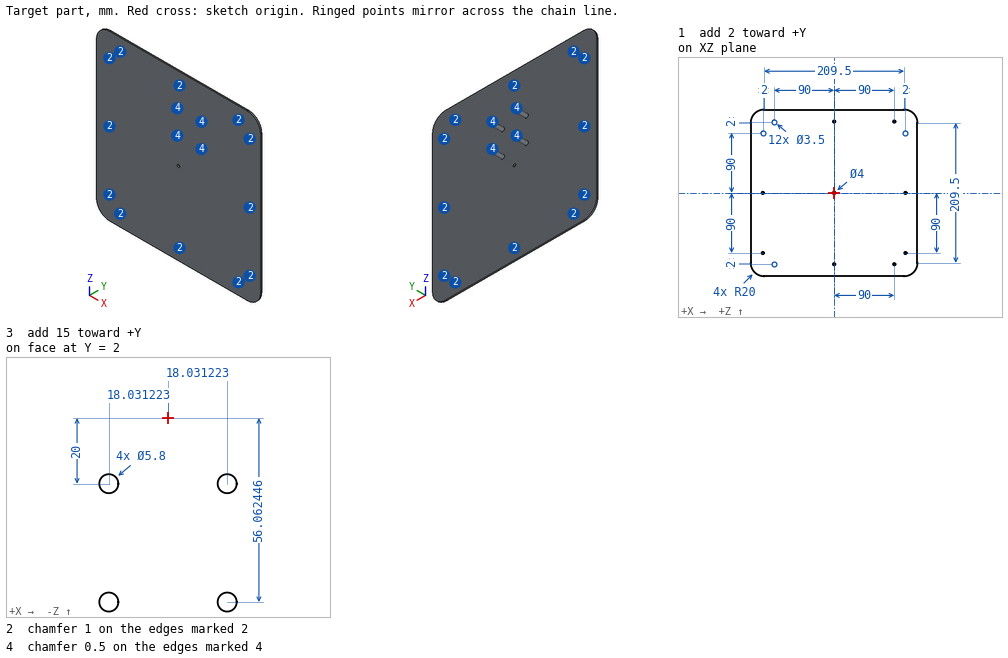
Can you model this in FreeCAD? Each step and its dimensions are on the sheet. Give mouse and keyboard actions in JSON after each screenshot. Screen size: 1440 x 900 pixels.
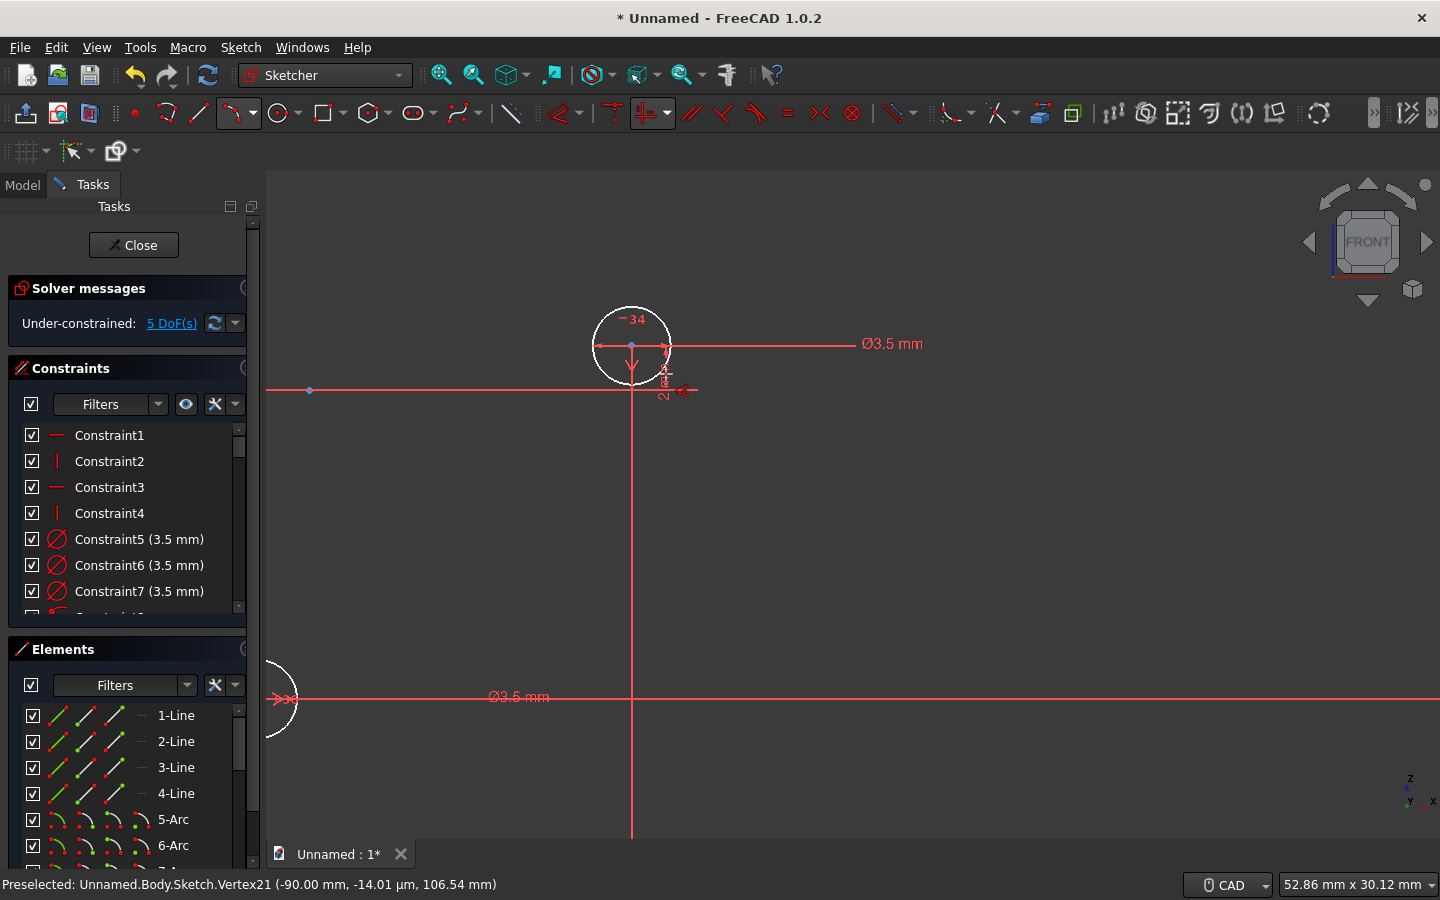
{"action": "scroll", "coordinate": [636, 328], "scroll_direction": "down", "scroll_amount": 13}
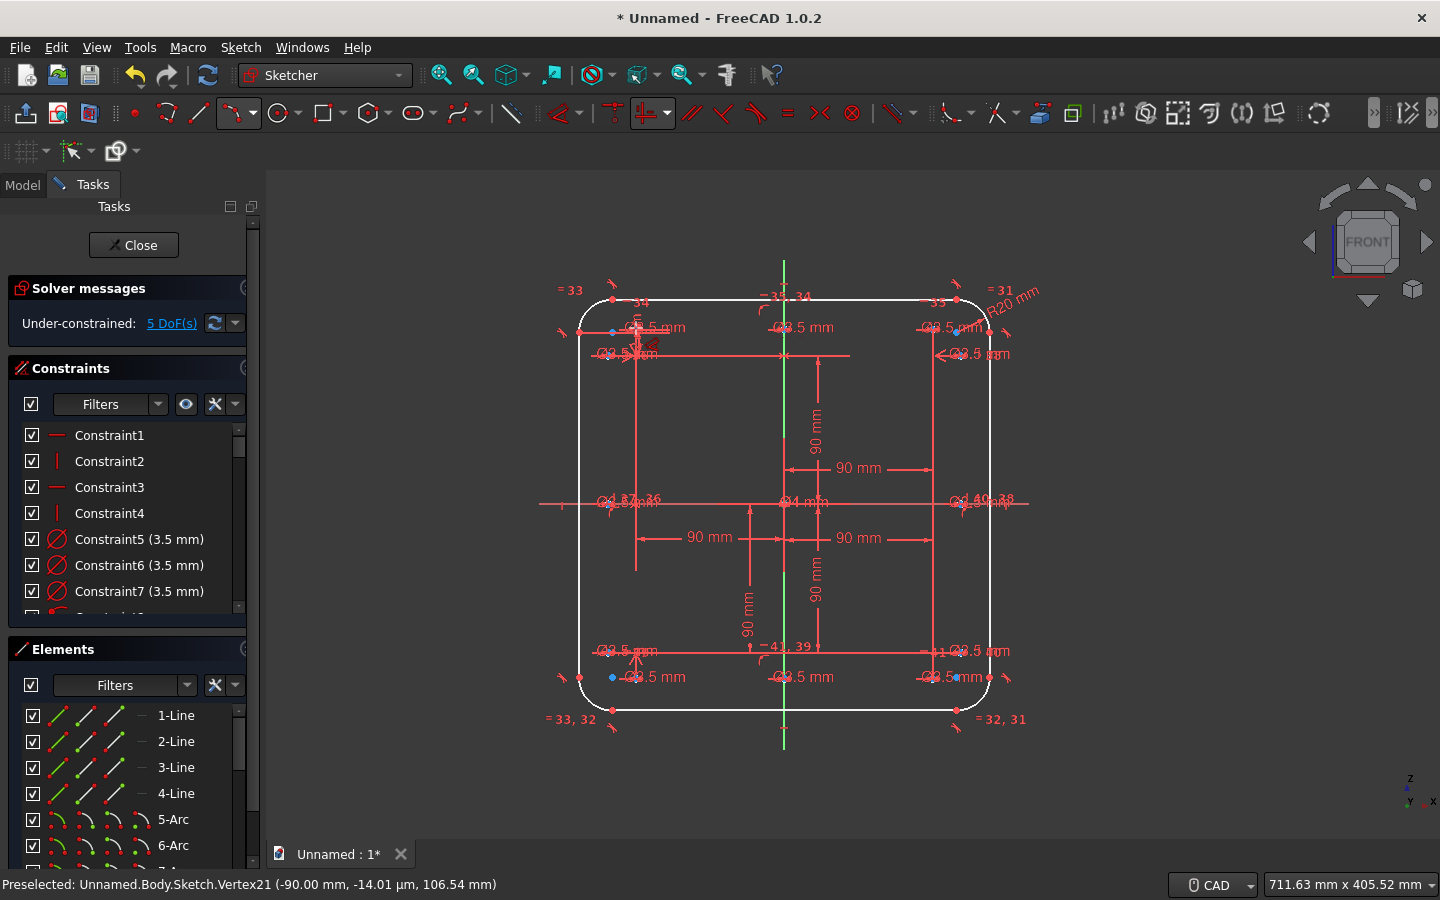
{"action": "scroll", "coordinate": [612, 300], "scroll_direction": "up", "scroll_amount": 13}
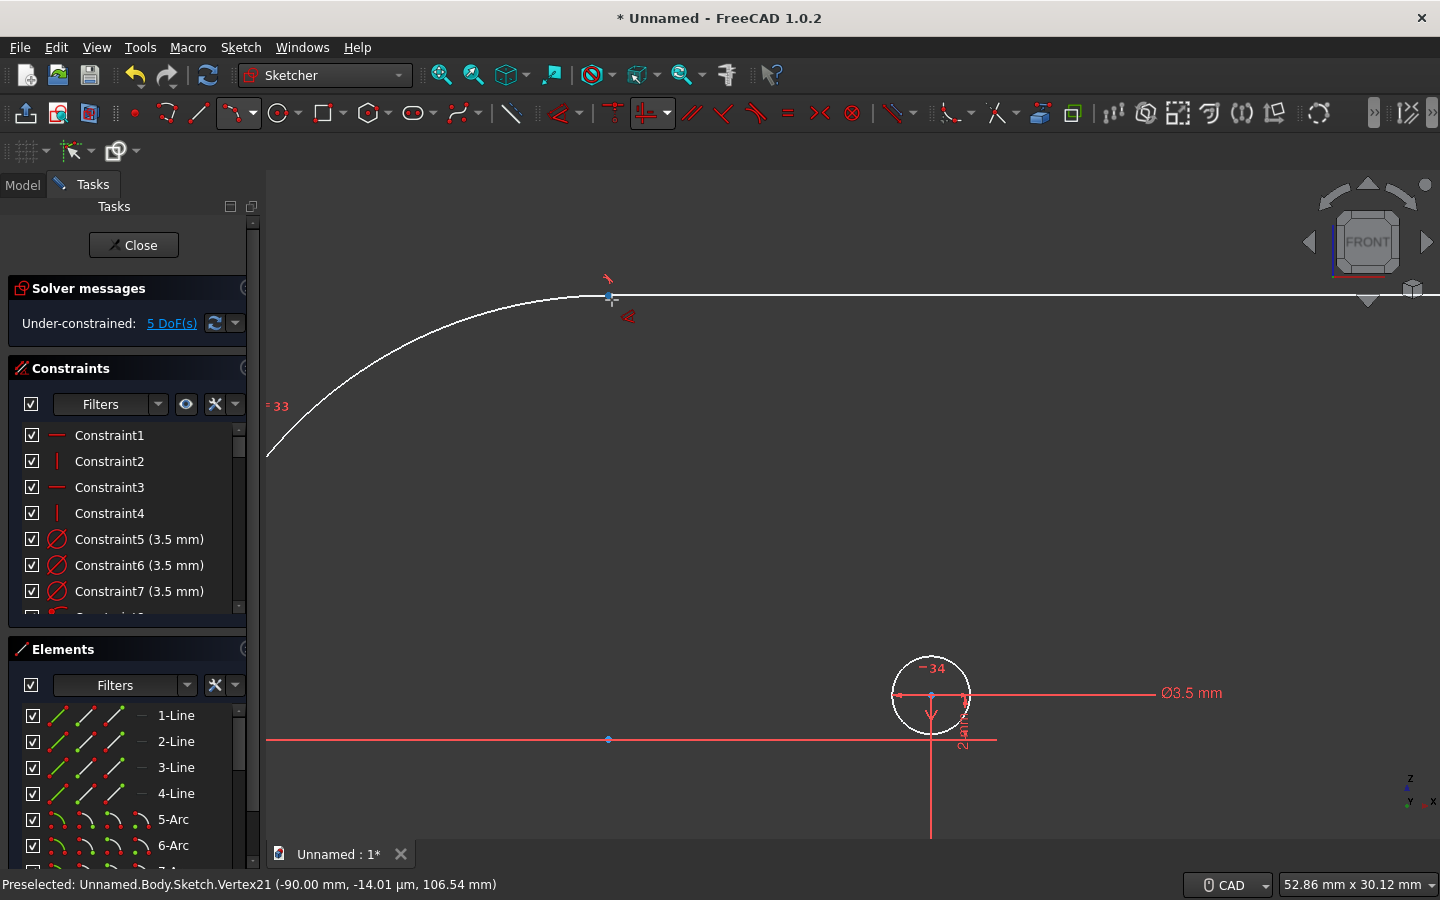
{"action": "left_click", "coordinate": [609, 295]}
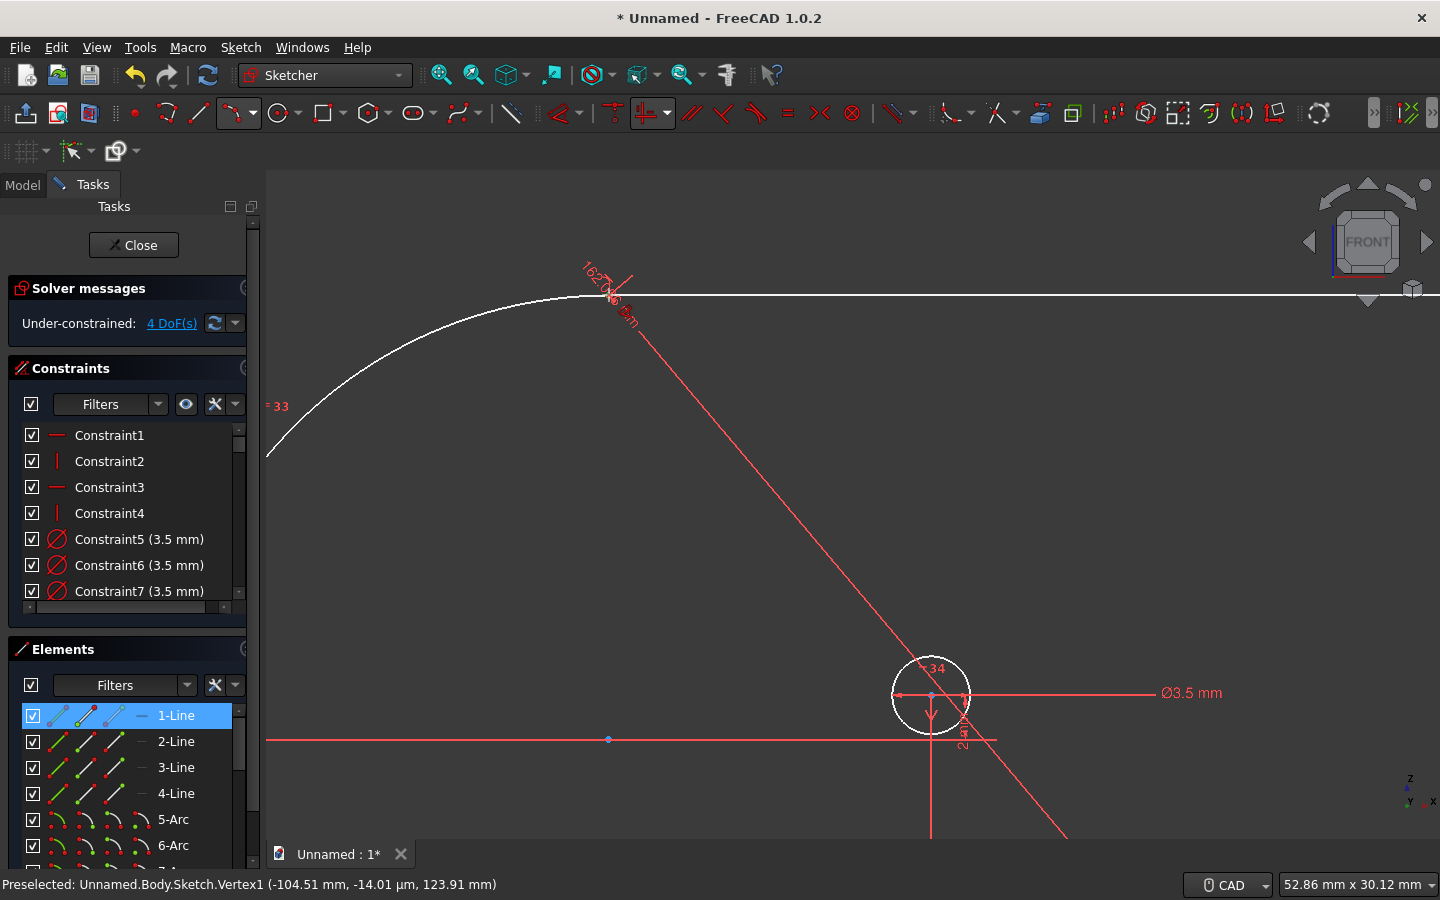
{"action": "scroll", "coordinate": [612, 300], "scroll_direction": "down", "scroll_amount": 13}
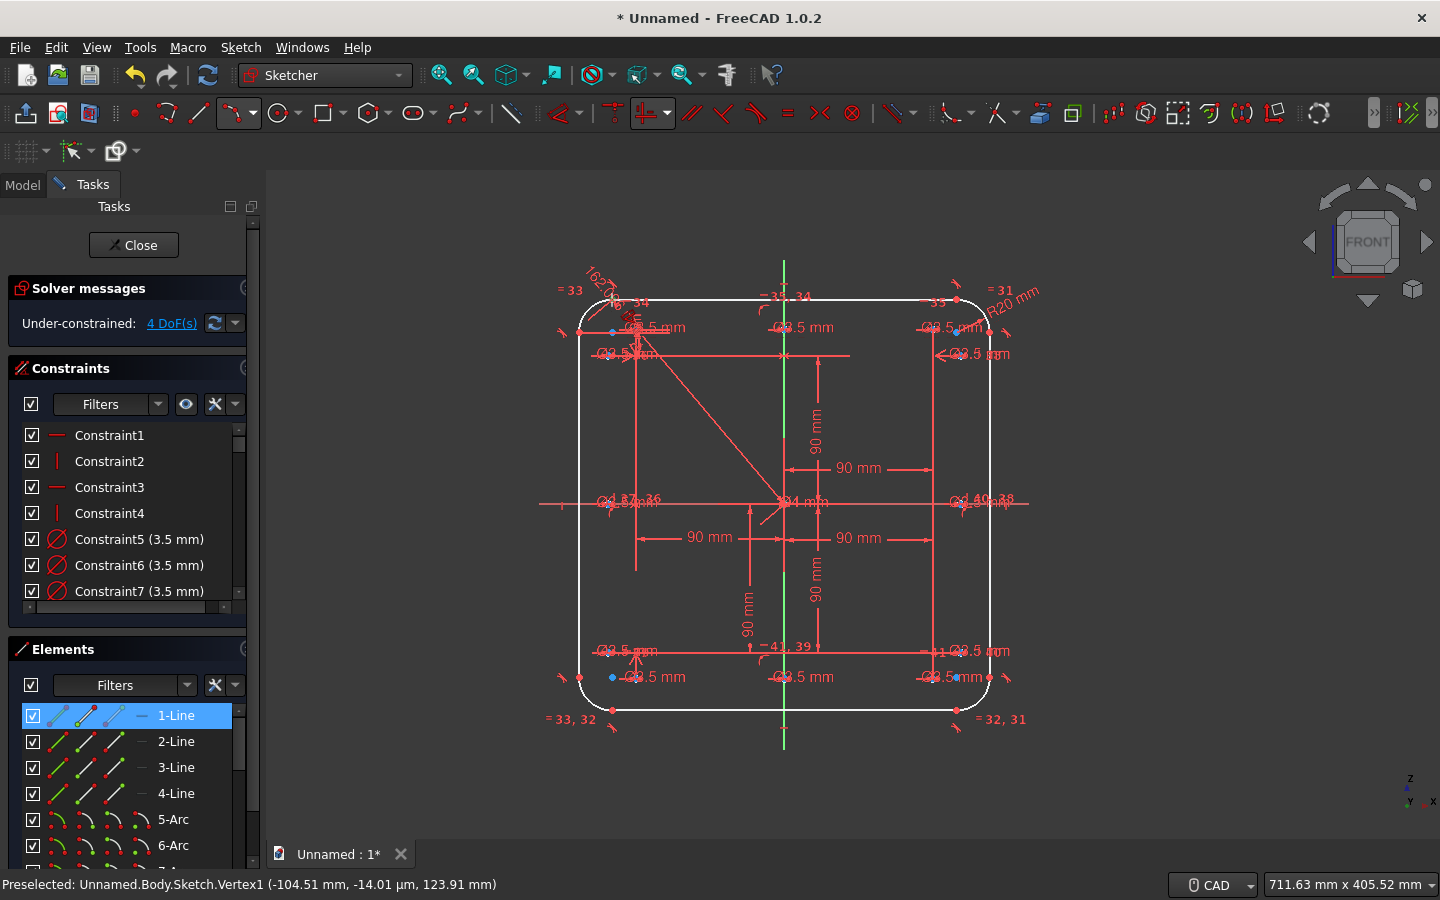
{"action": "scroll", "coordinate": [608, 356], "scroll_direction": "up", "scroll_amount": 13}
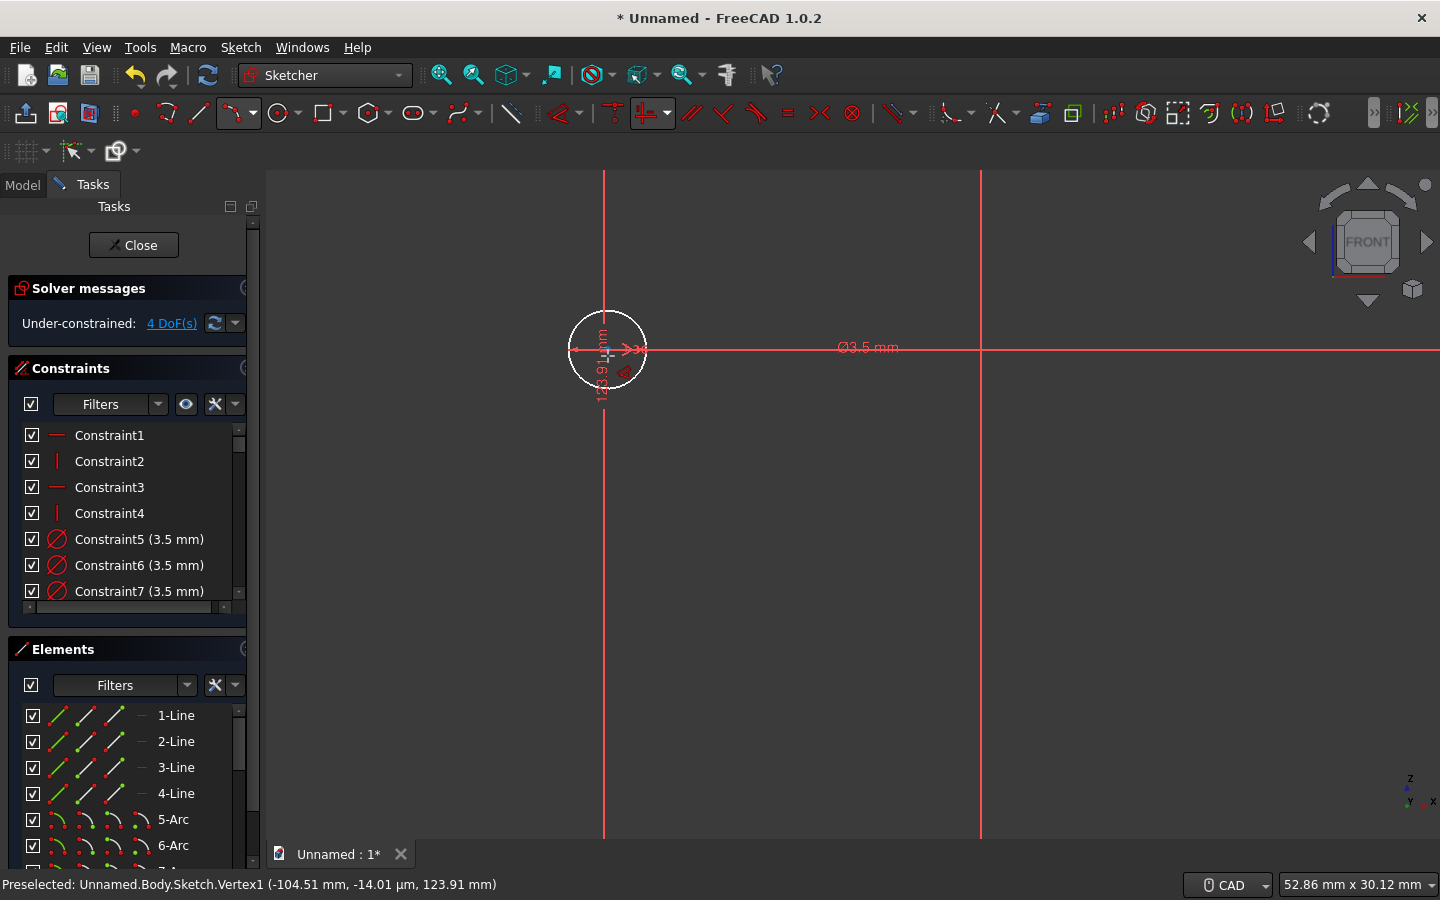
{"action": "left_click", "coordinate": [607, 350]}
{"action": "left_click", "coordinate": [651, 384]}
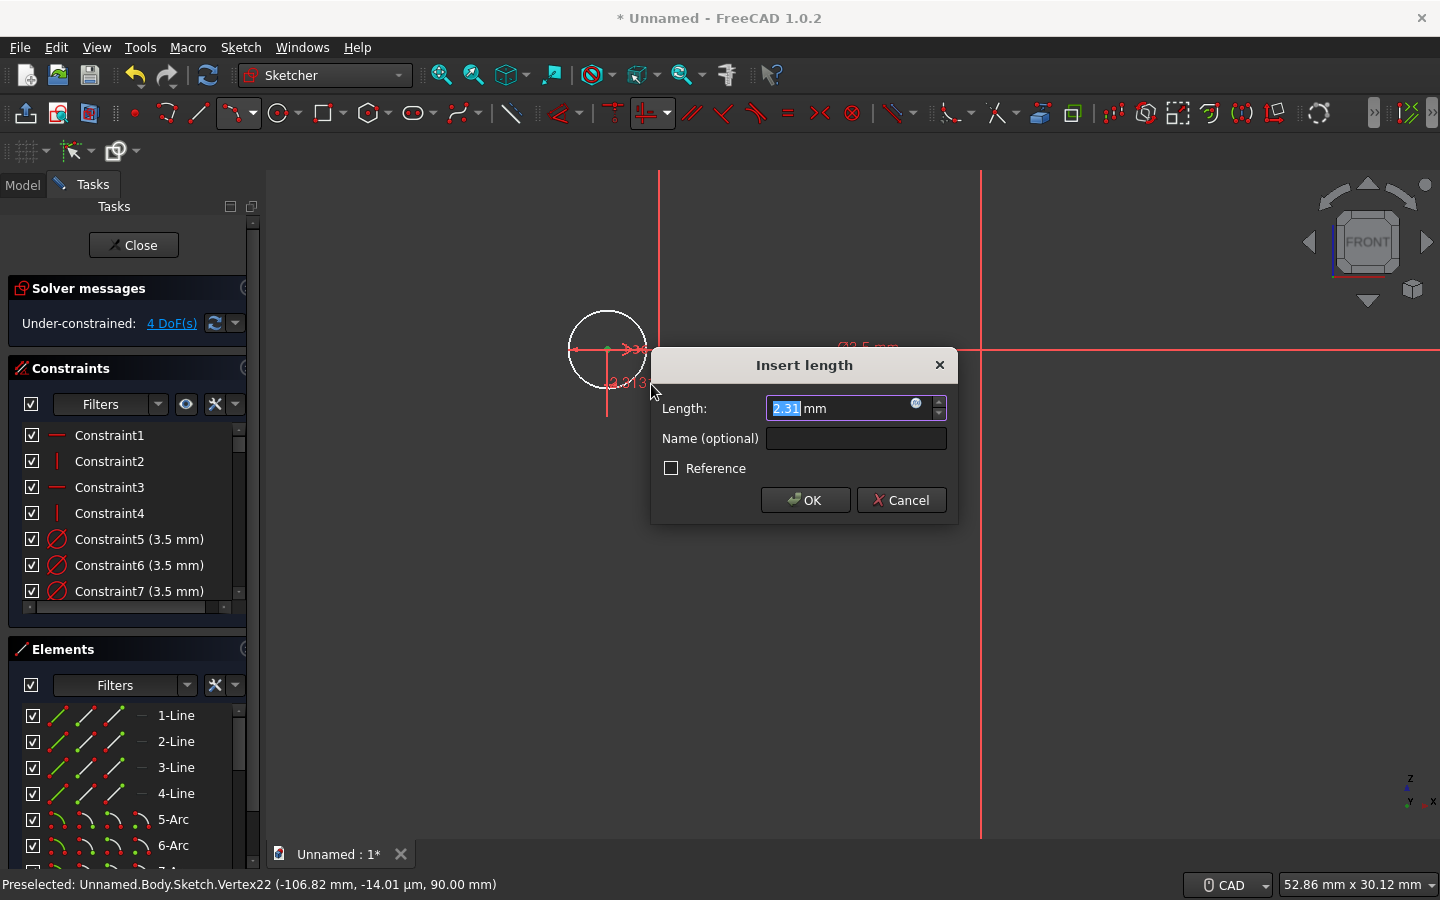
{"action": "type", "text": "2"}
{"action": "key", "text": "Return"}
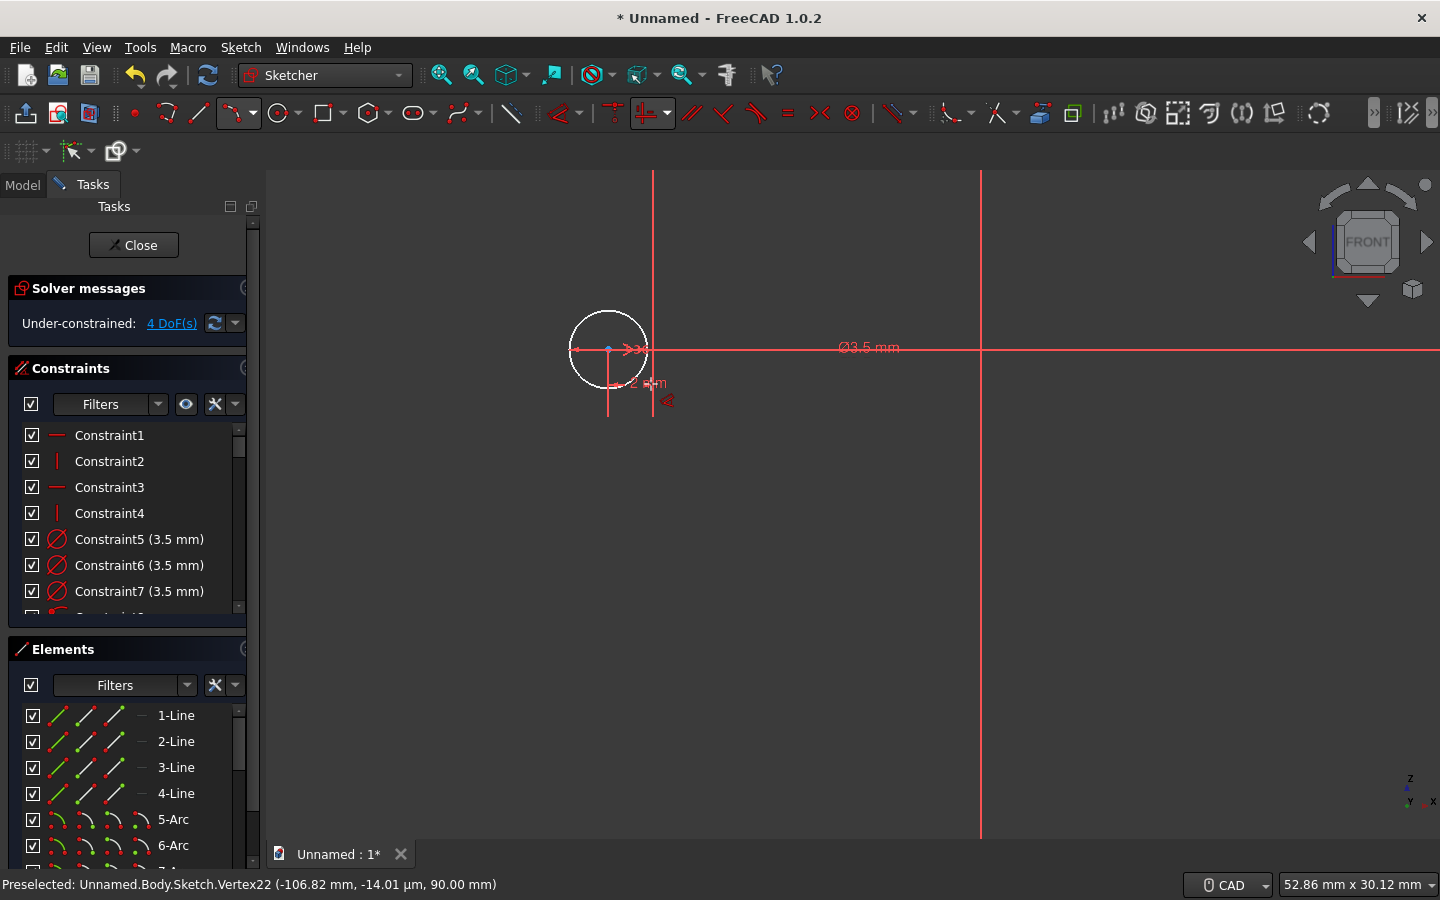
{"action": "scroll", "coordinate": [608, 357], "scroll_direction": "down", "scroll_amount": 13}